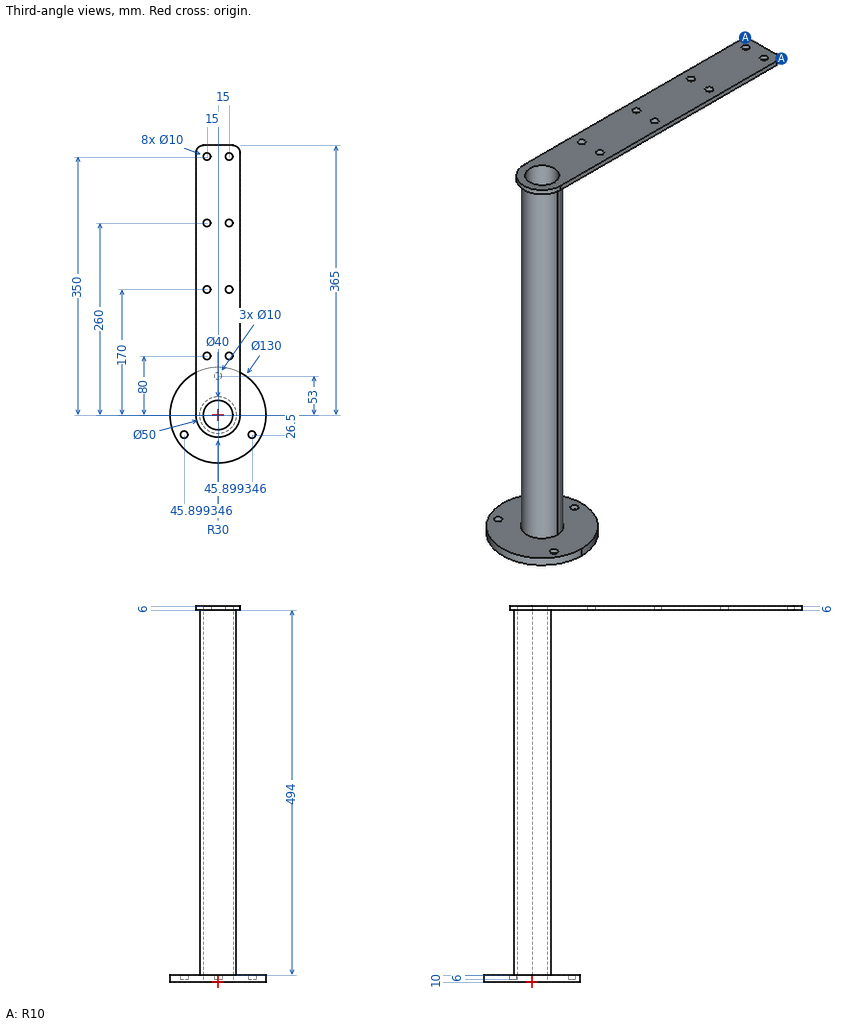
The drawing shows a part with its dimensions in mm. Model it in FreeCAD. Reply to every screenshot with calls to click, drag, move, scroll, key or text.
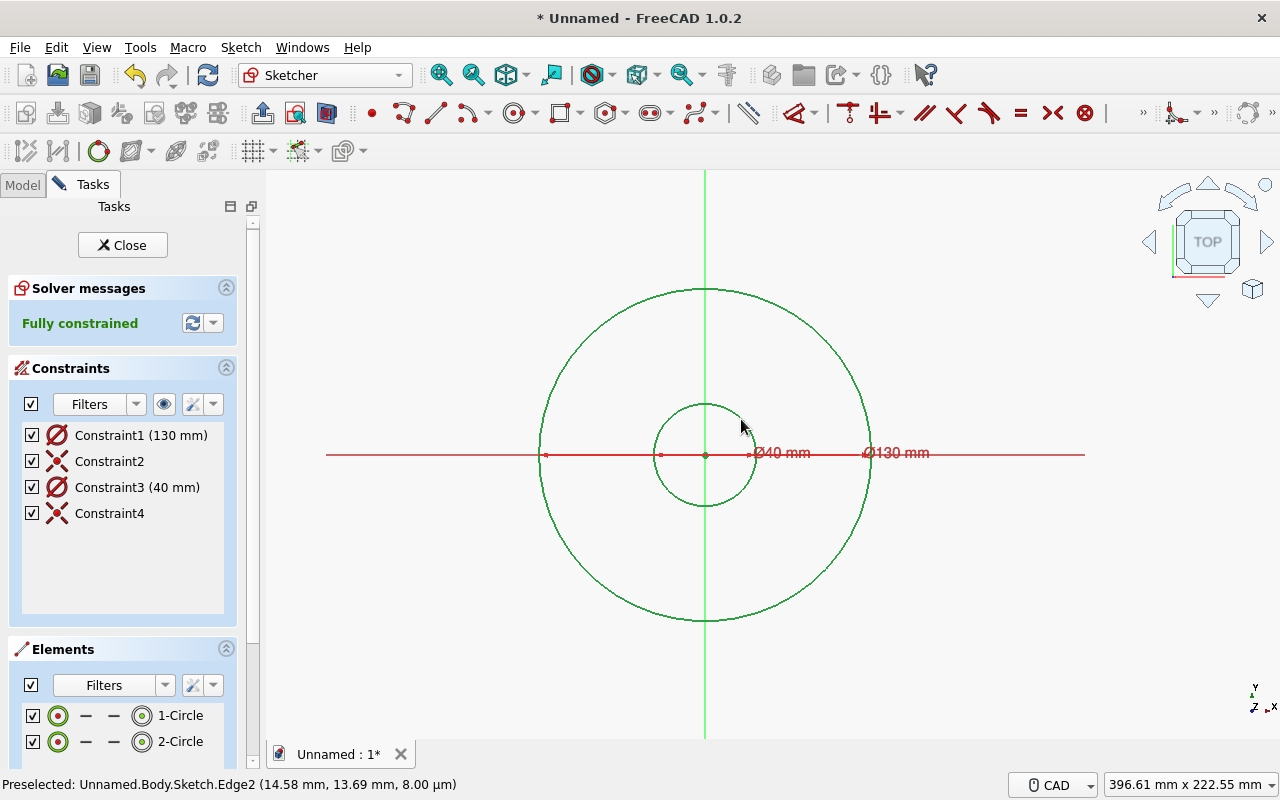
click(123, 245)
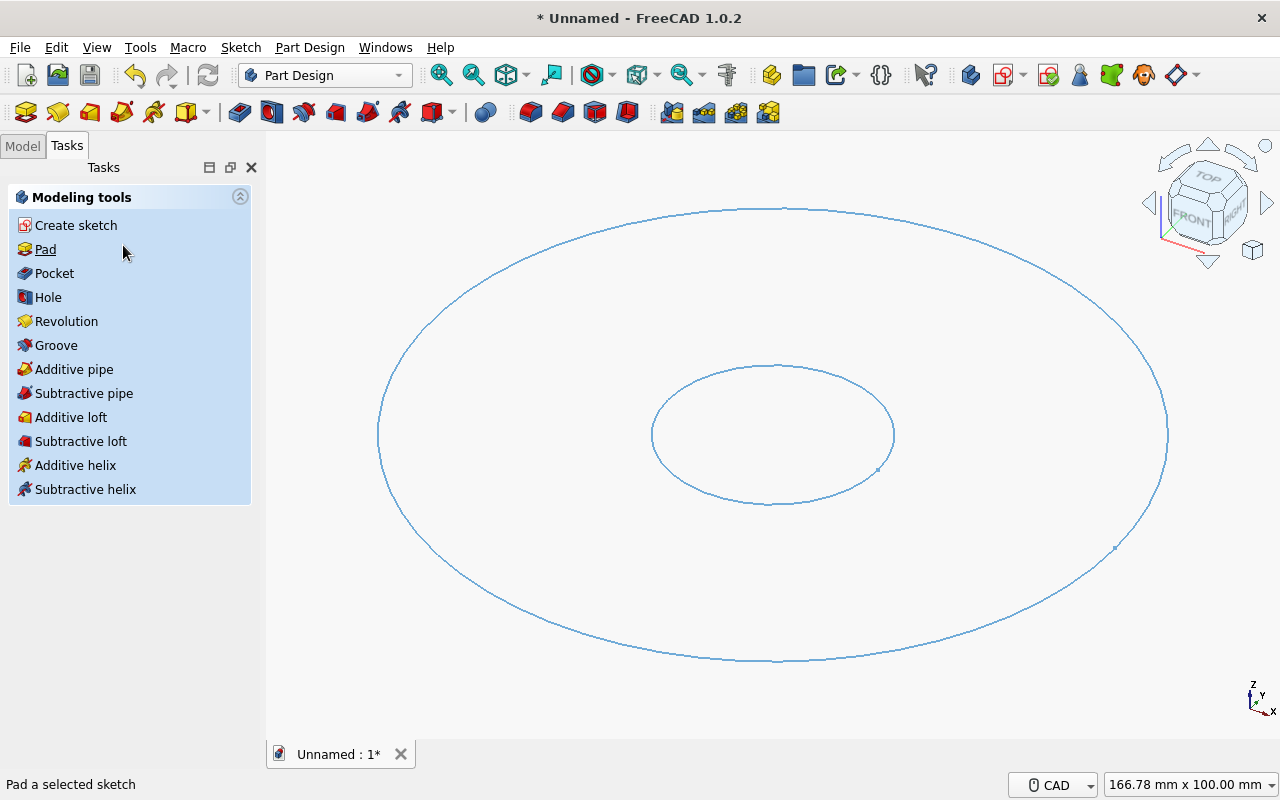
click(26, 112)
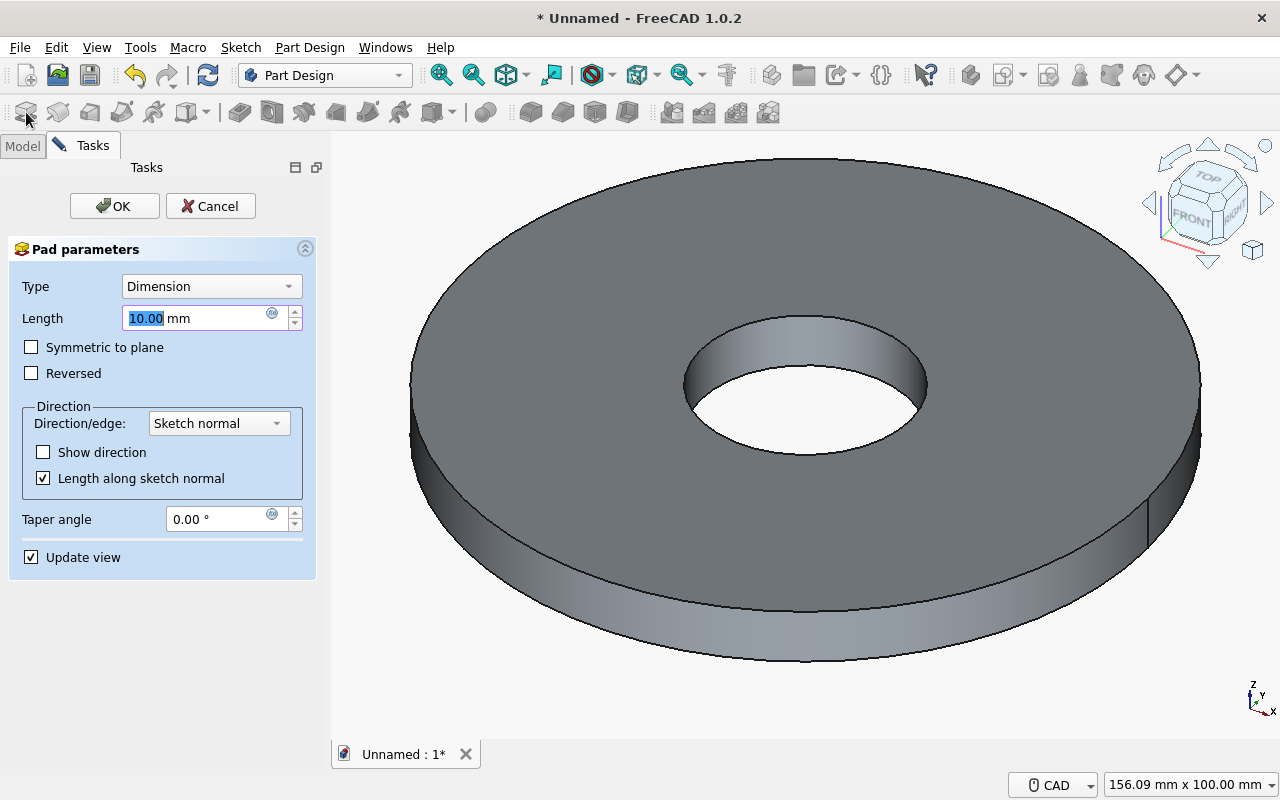
text(10)
key(Tab)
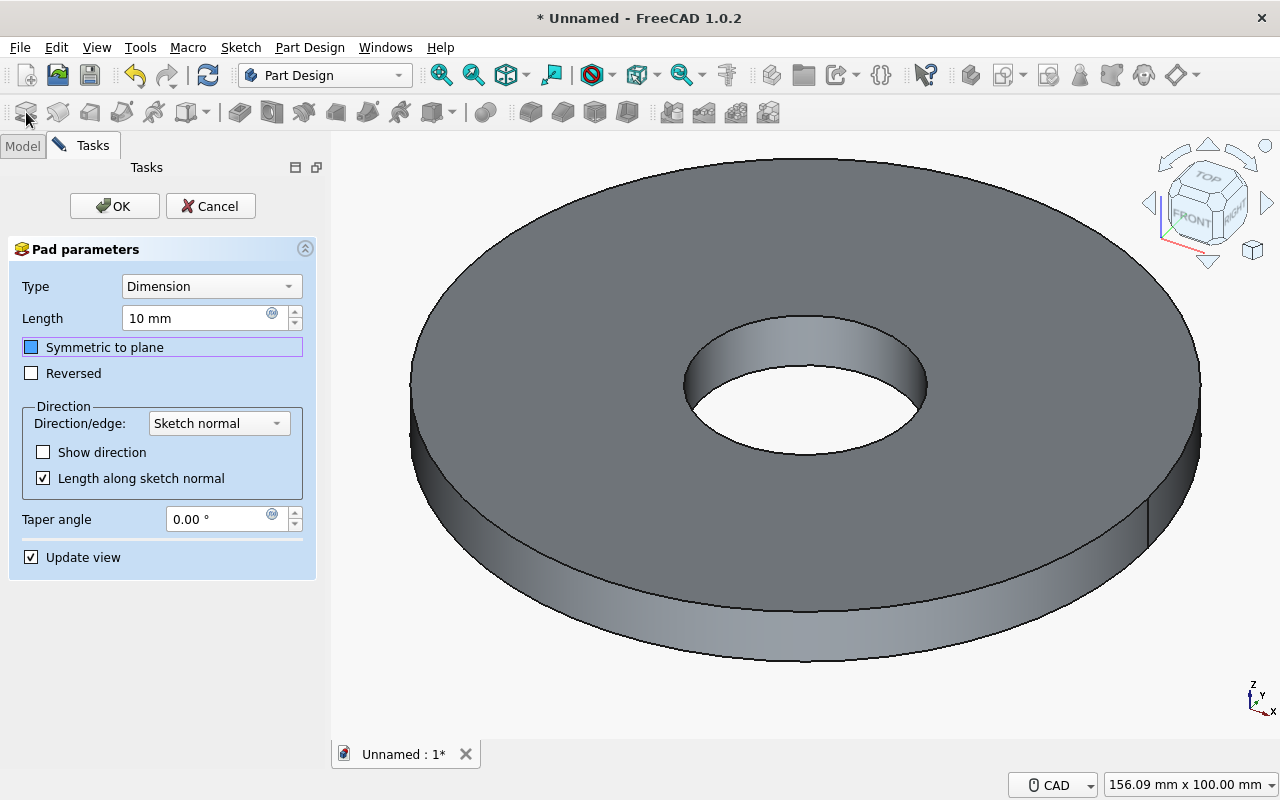
click(115, 206)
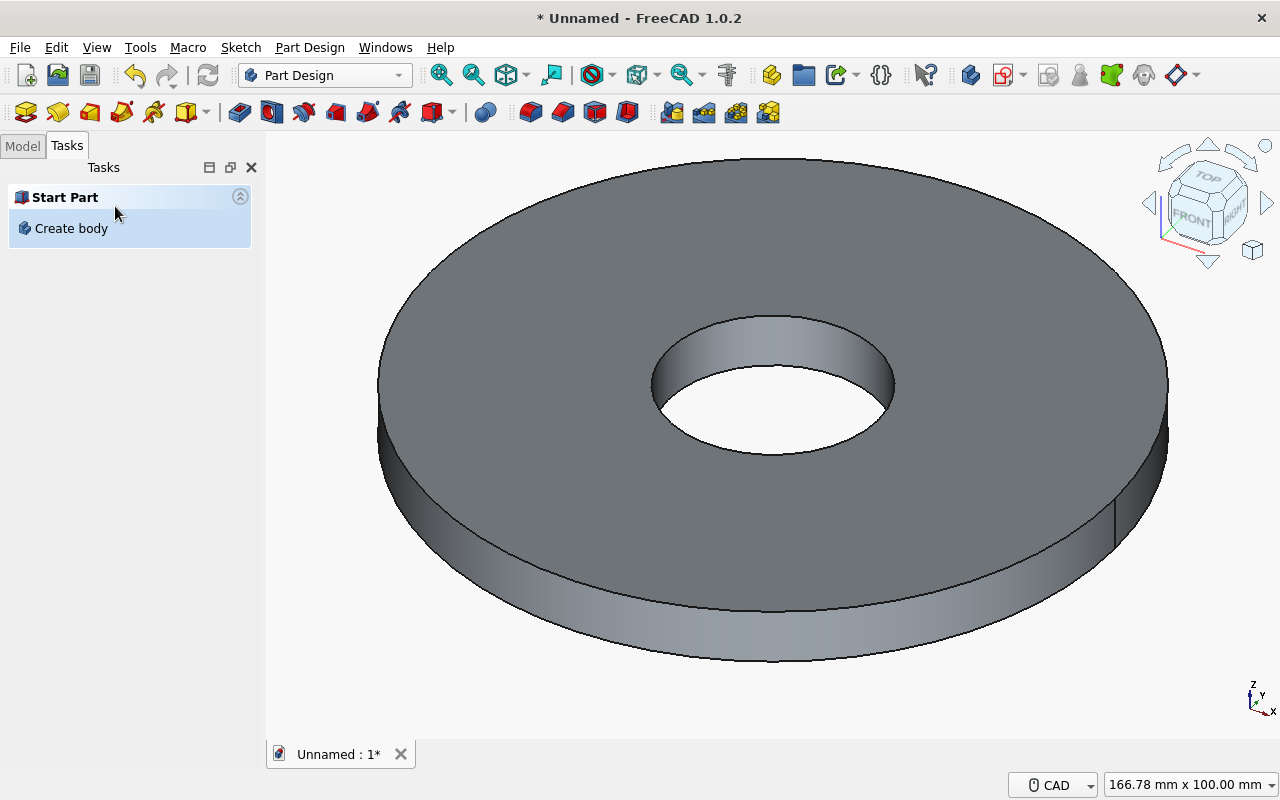
click(442, 76)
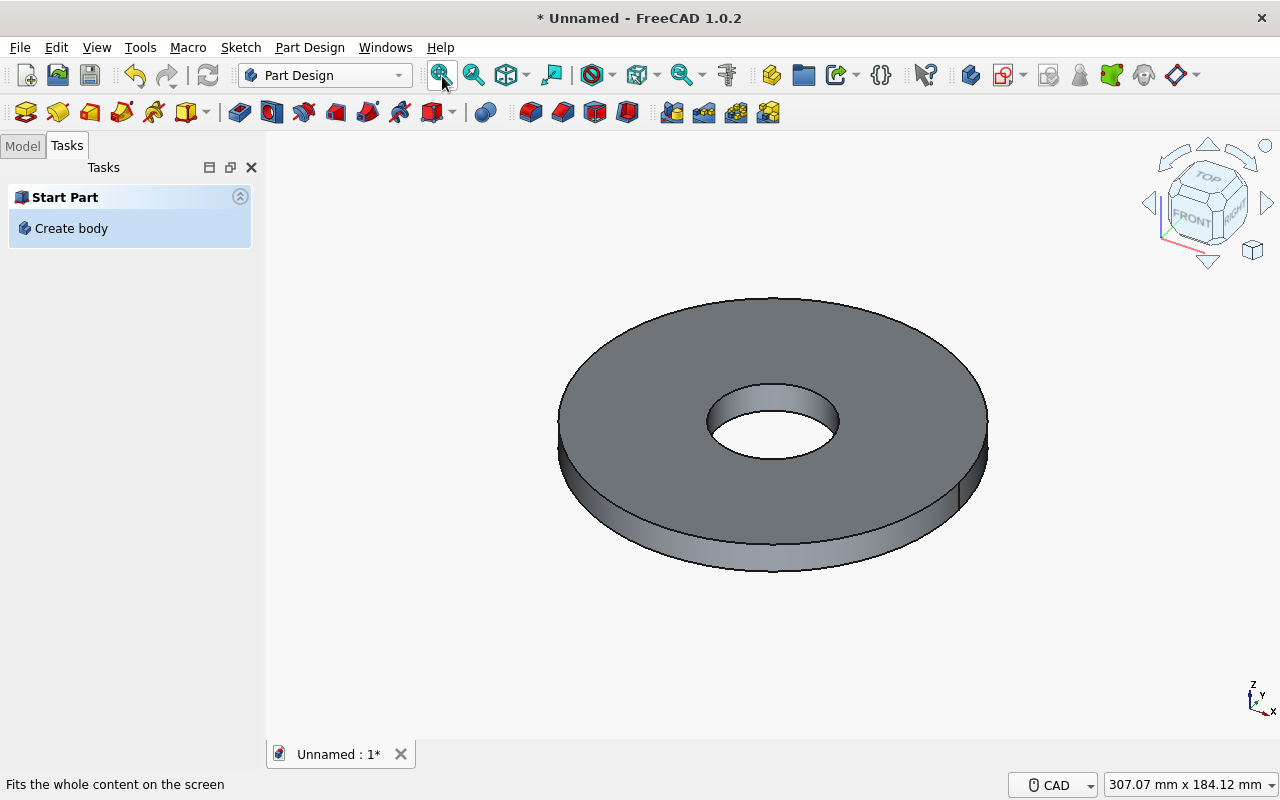
click(659, 464)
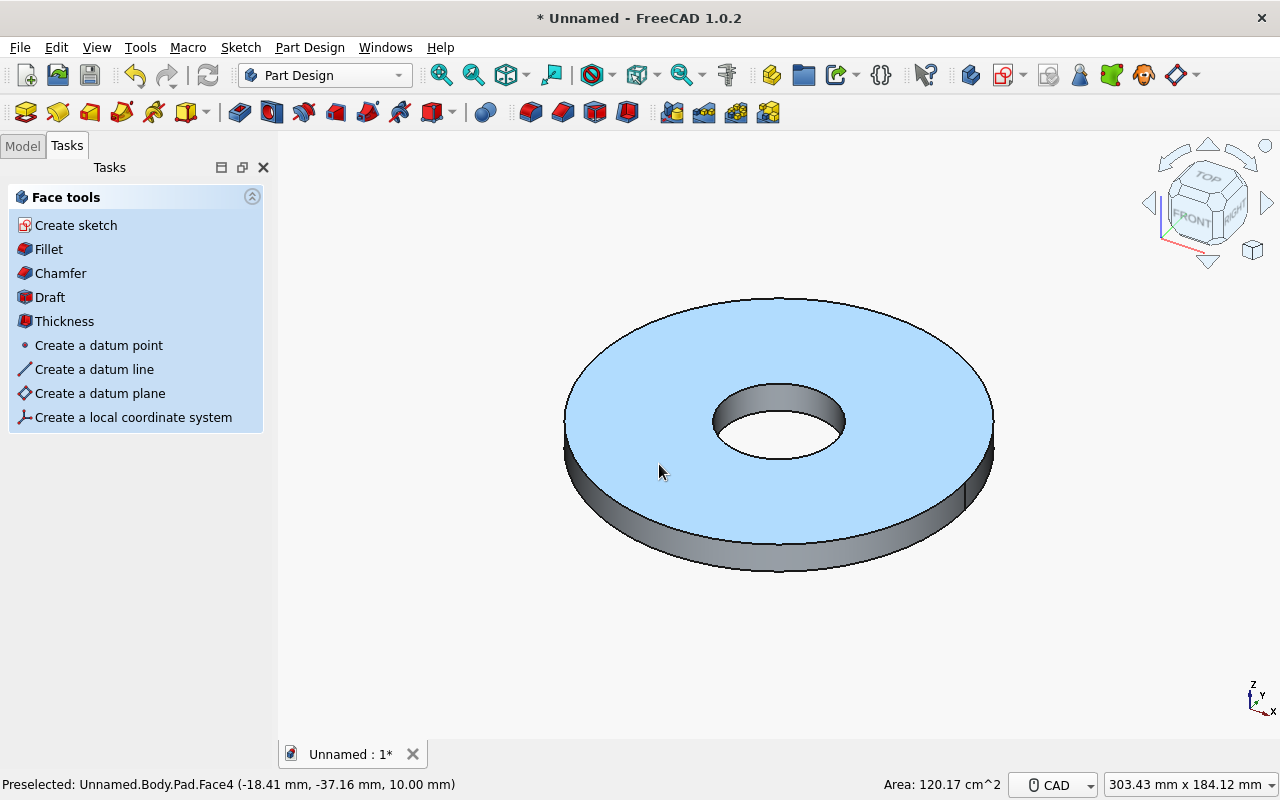
click(1004, 76)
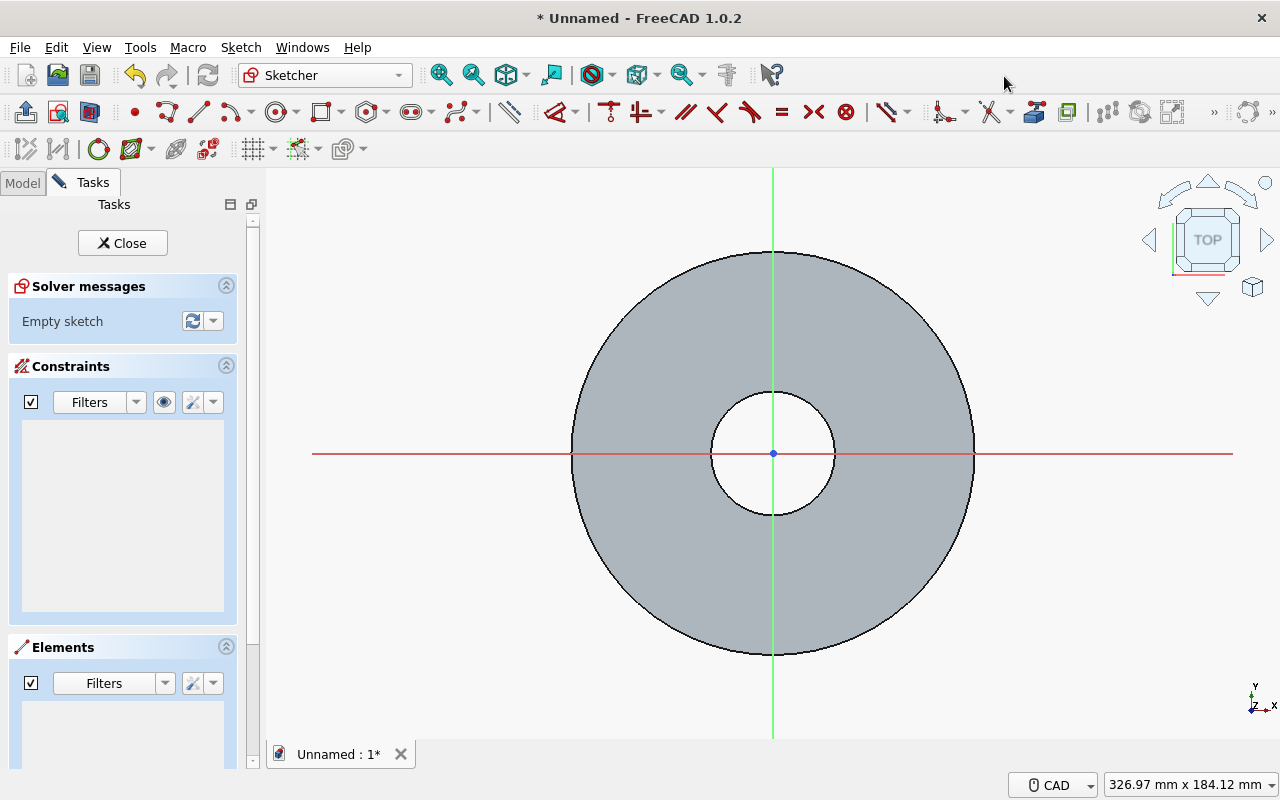
scroll(829, 454, up, 4)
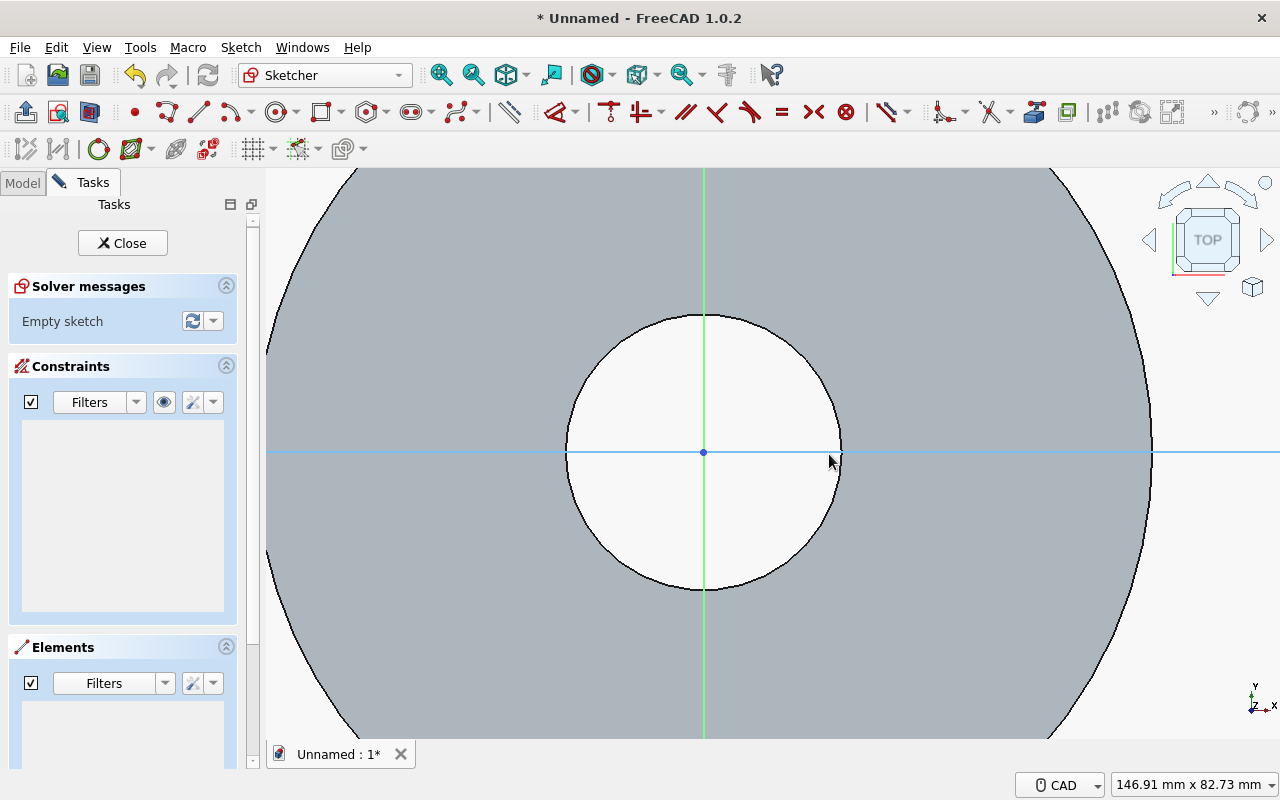
click(276, 112)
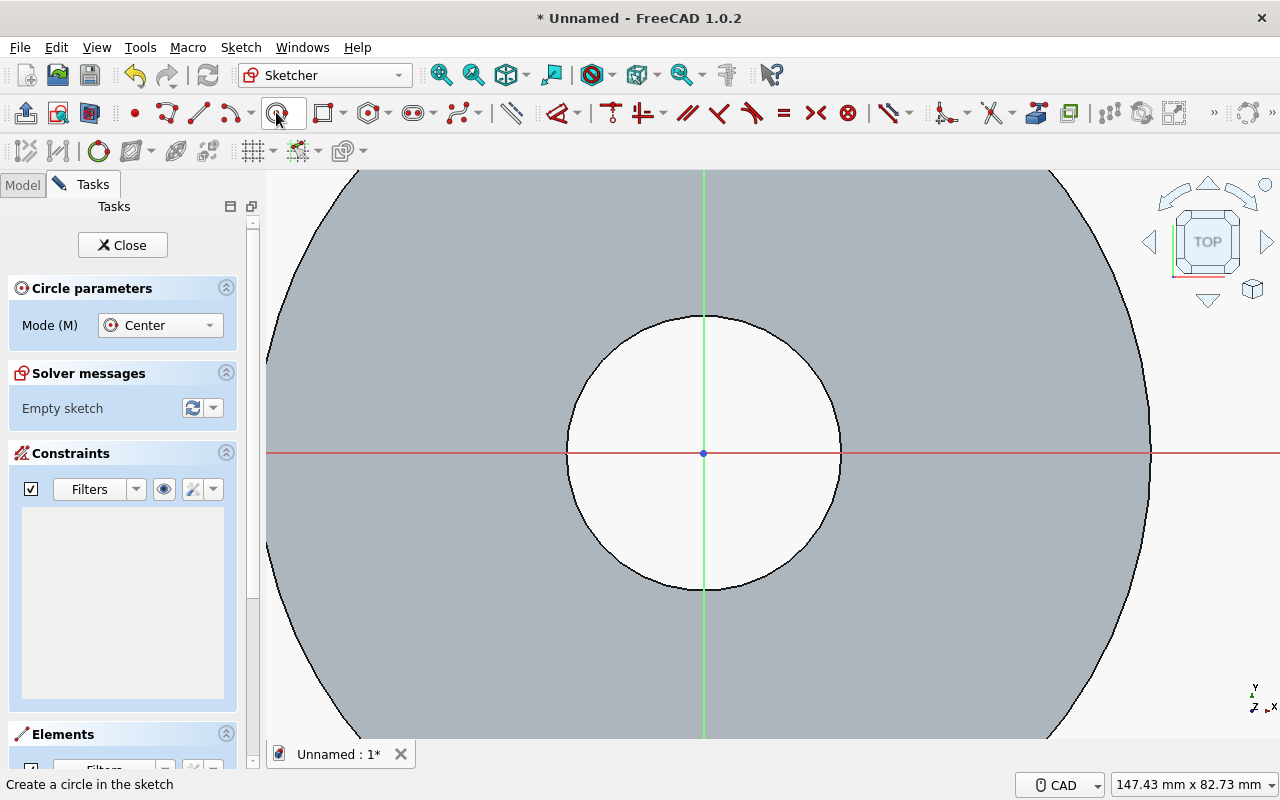
click(704, 453)
move(826, 332)